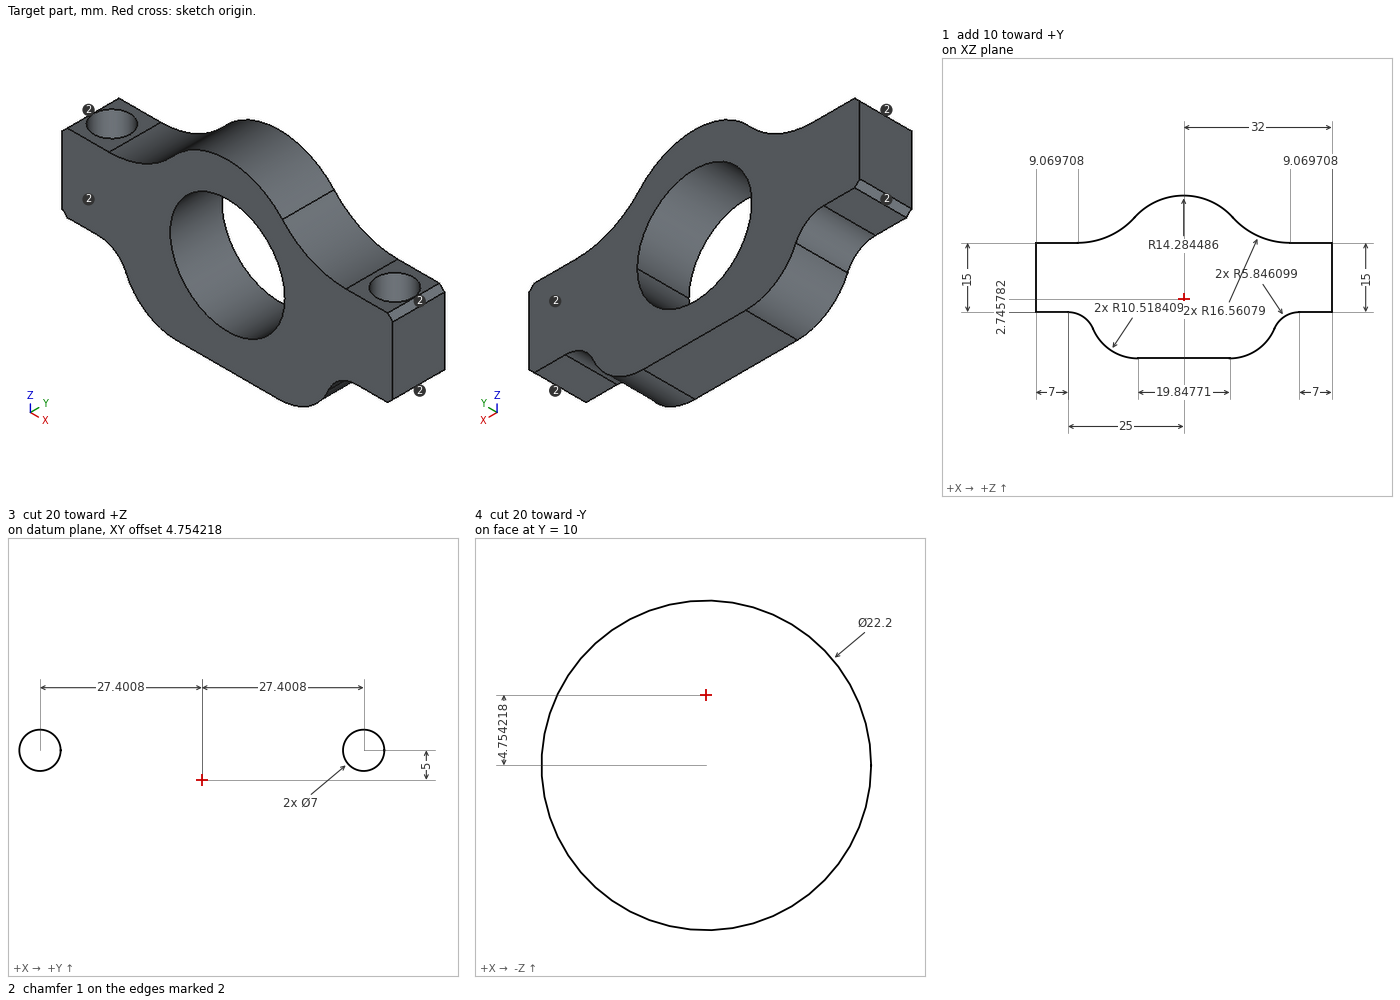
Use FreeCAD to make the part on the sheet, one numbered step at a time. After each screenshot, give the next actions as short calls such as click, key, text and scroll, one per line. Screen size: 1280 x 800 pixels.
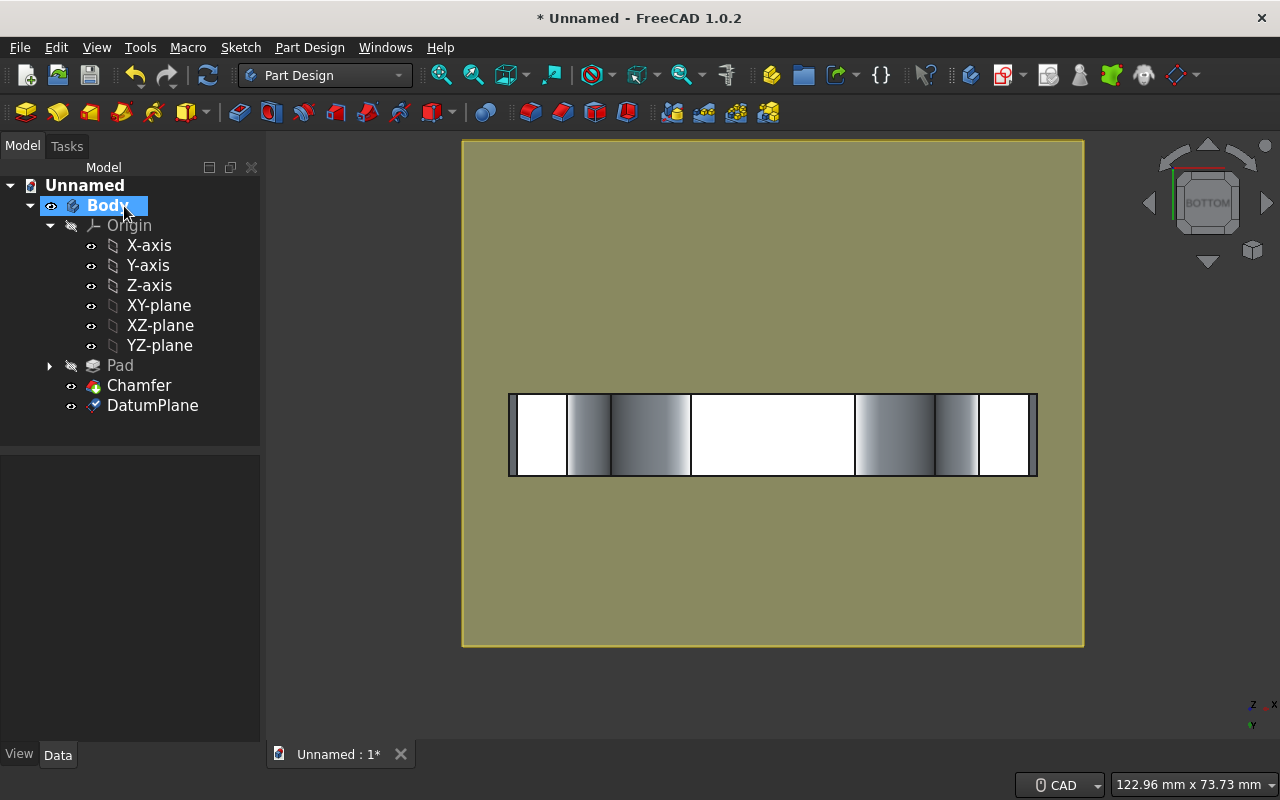
click(116, 406)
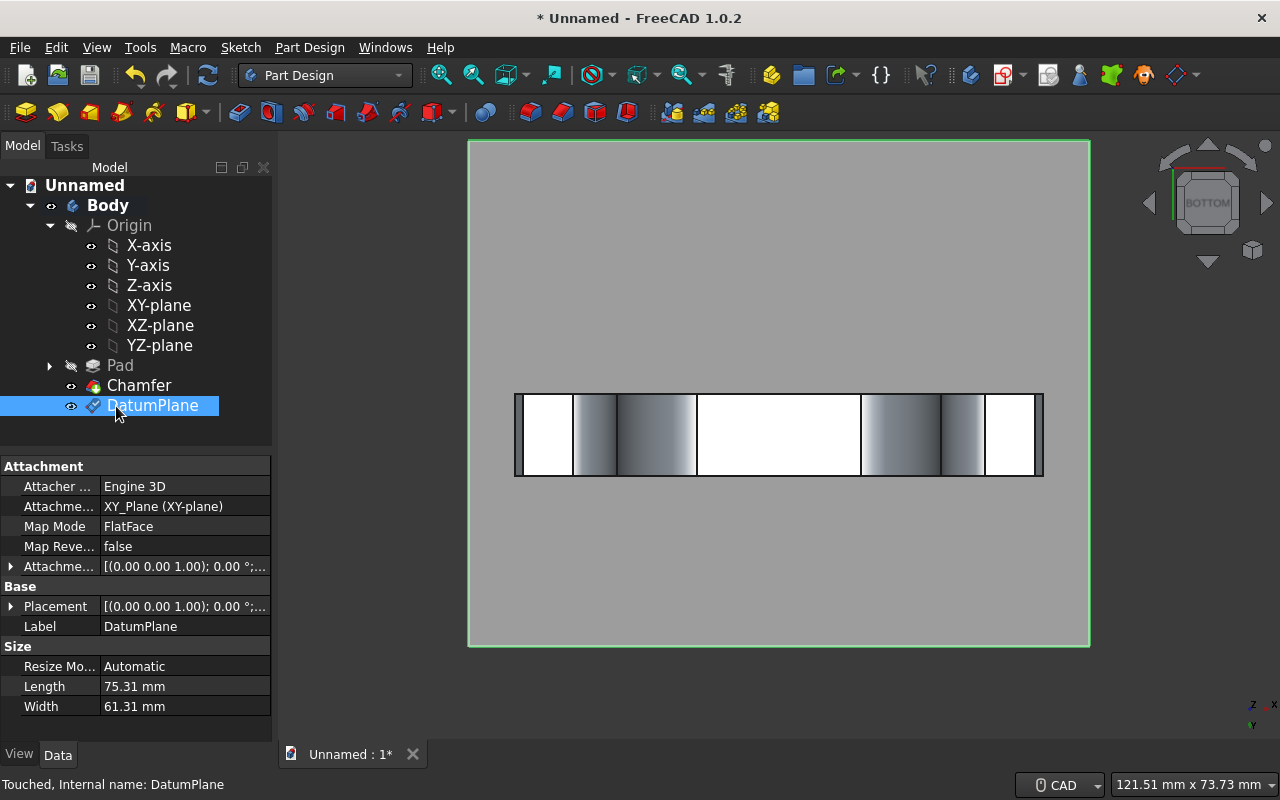
click(1004, 76)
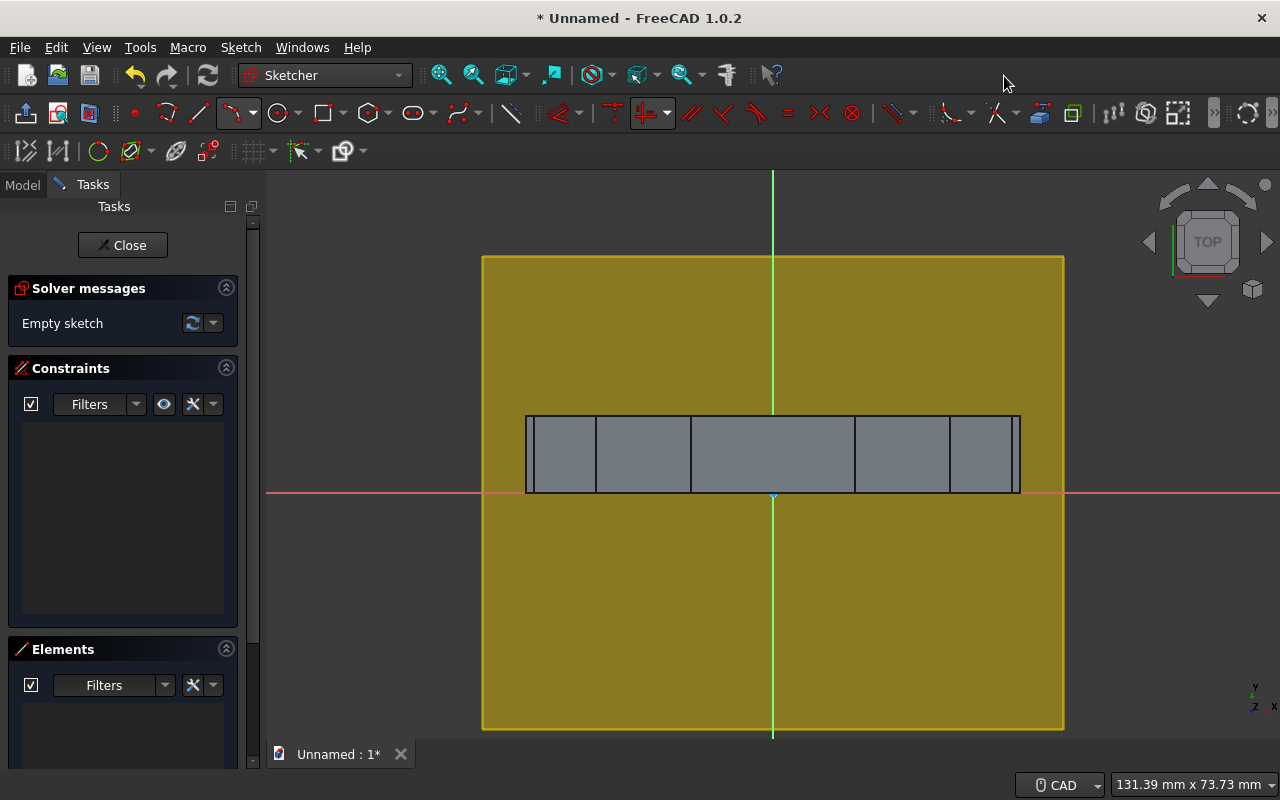
click(90, 114)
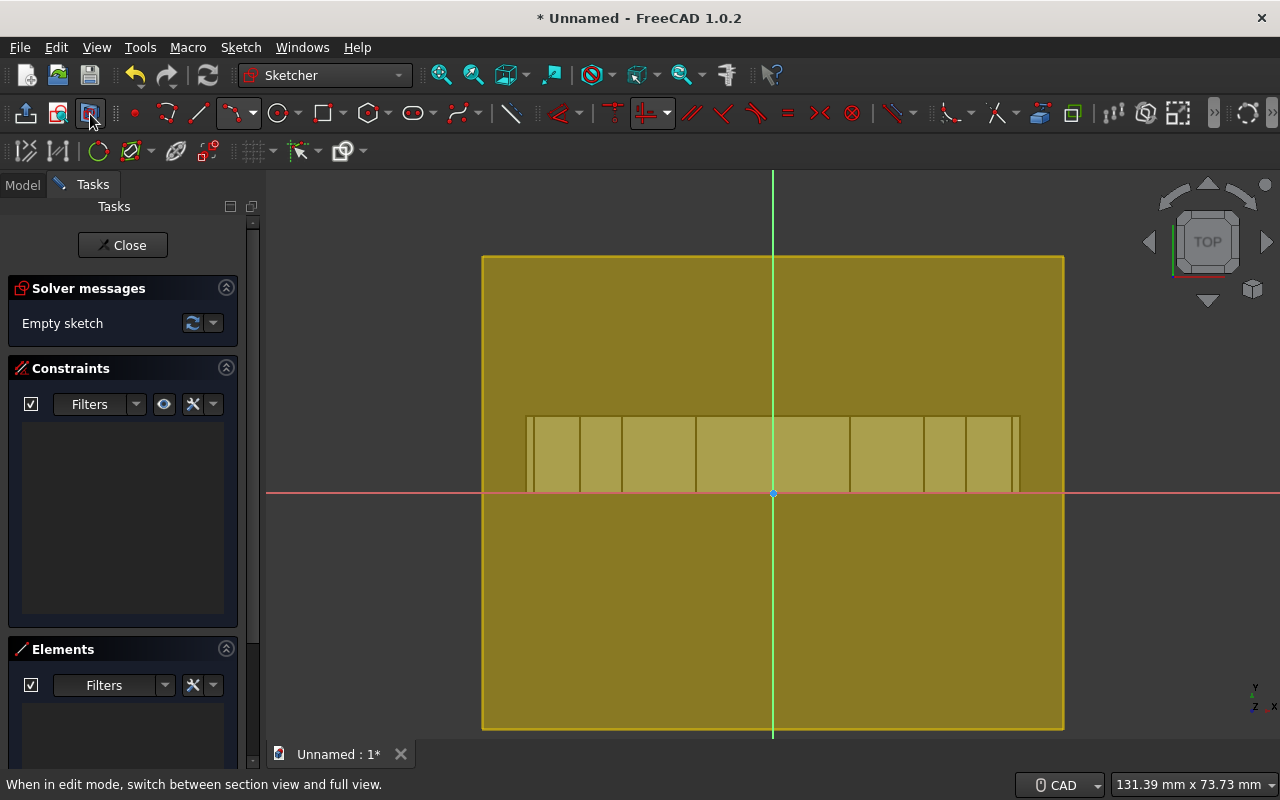
click(278, 114)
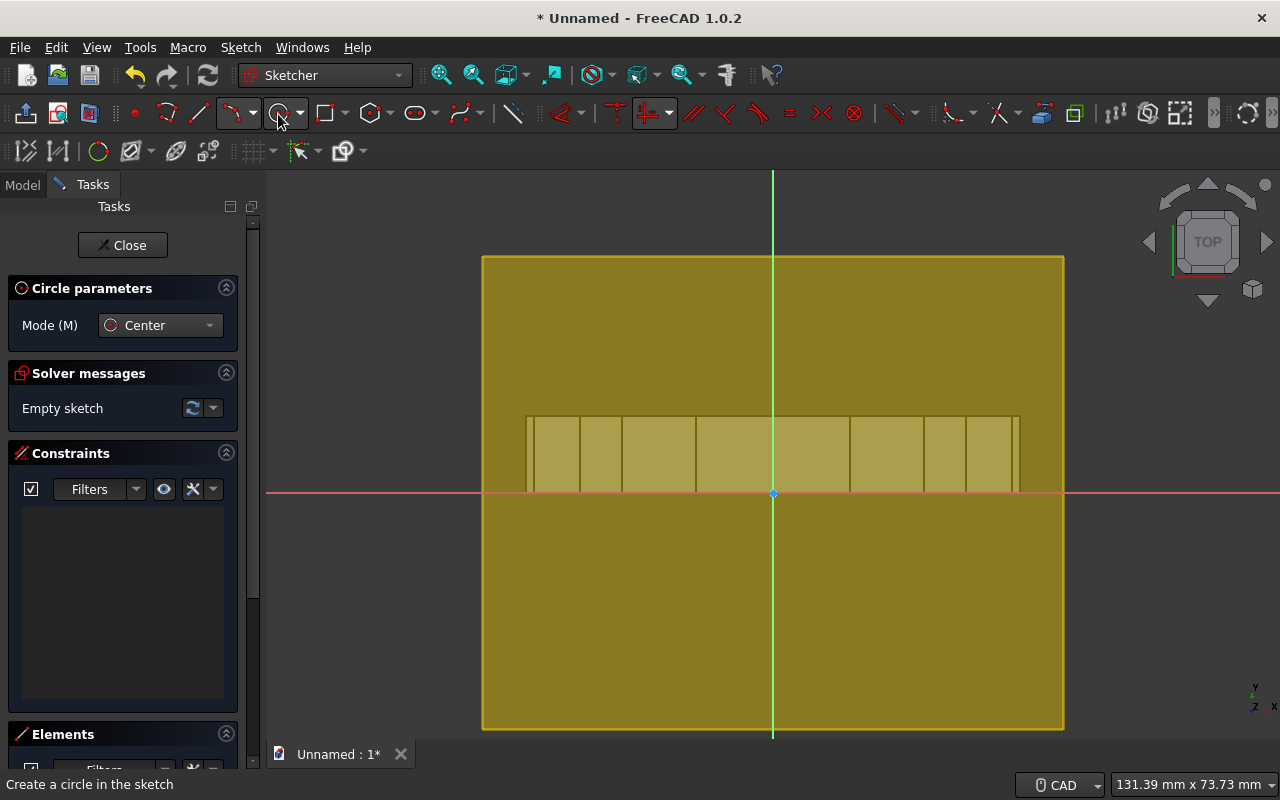
click(984, 454)
move(1004, 435)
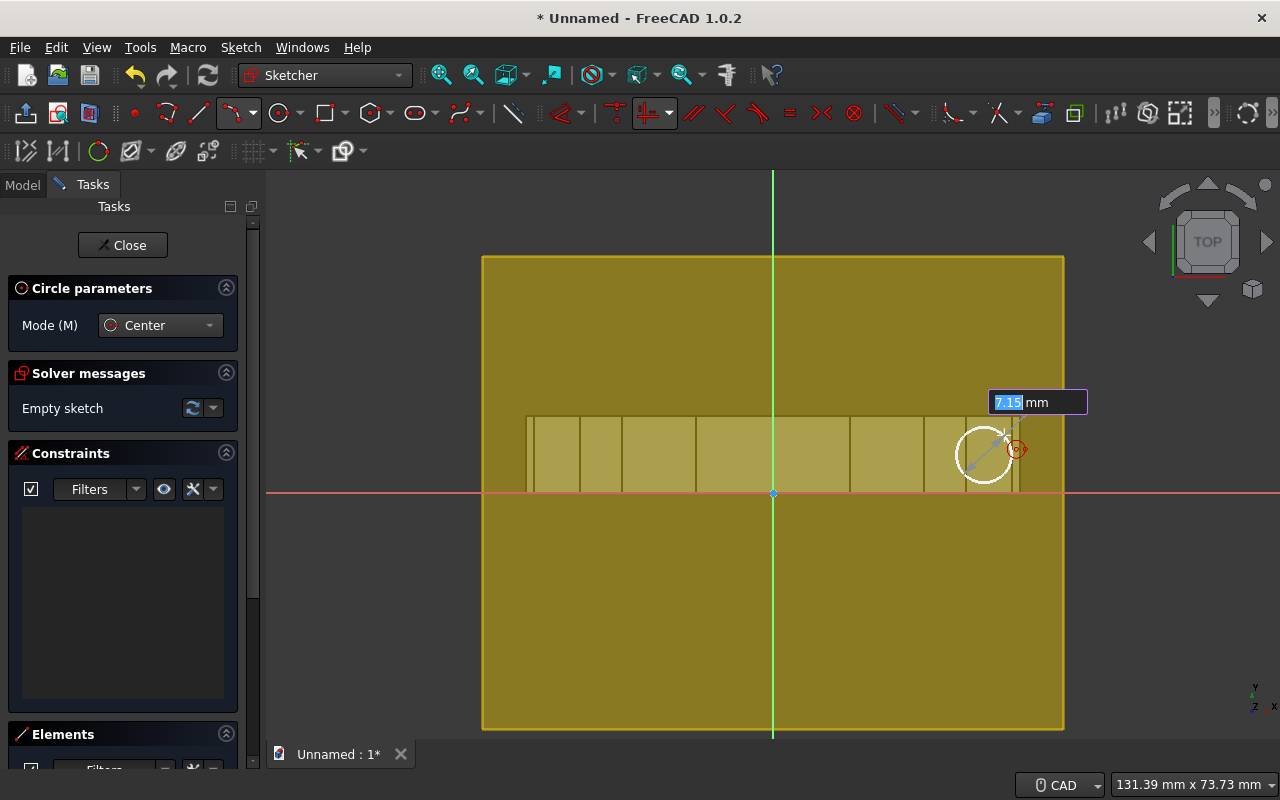
text(7)
key(Return)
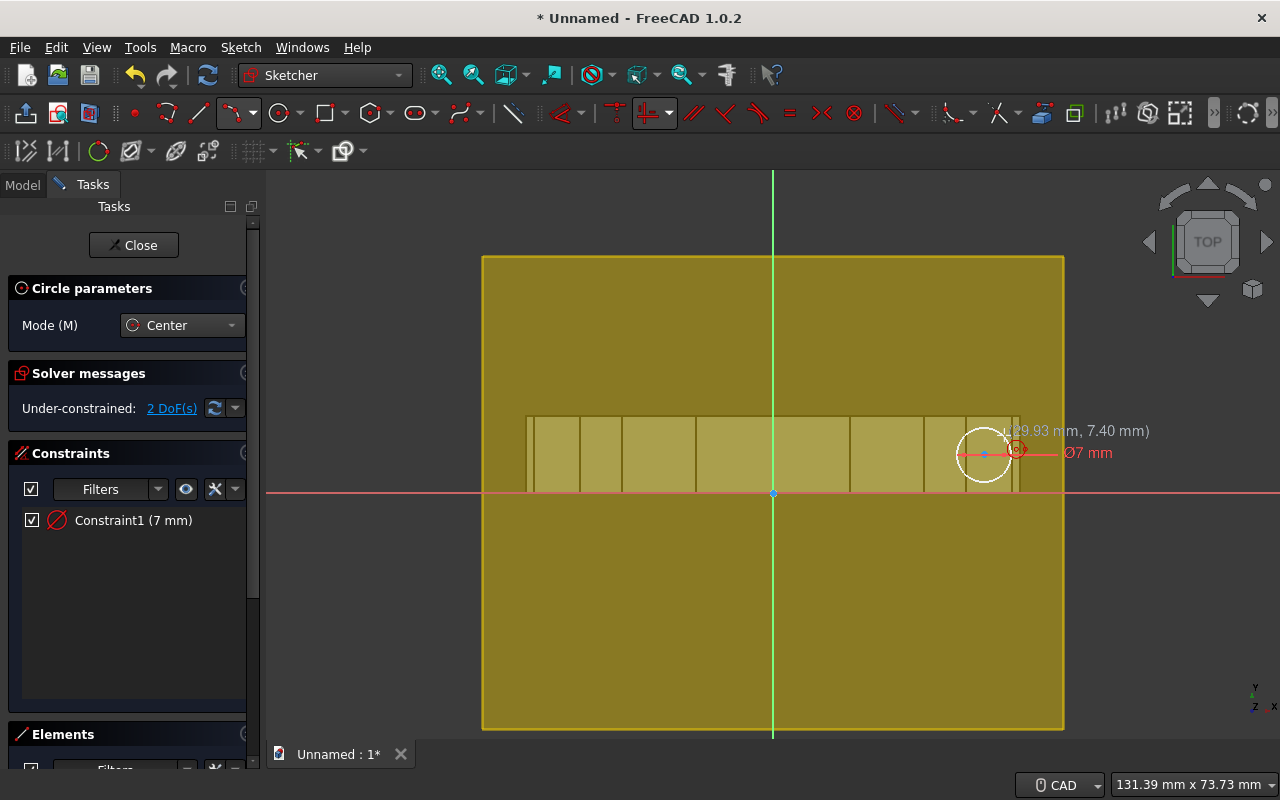
click(562, 454)
move(581, 435)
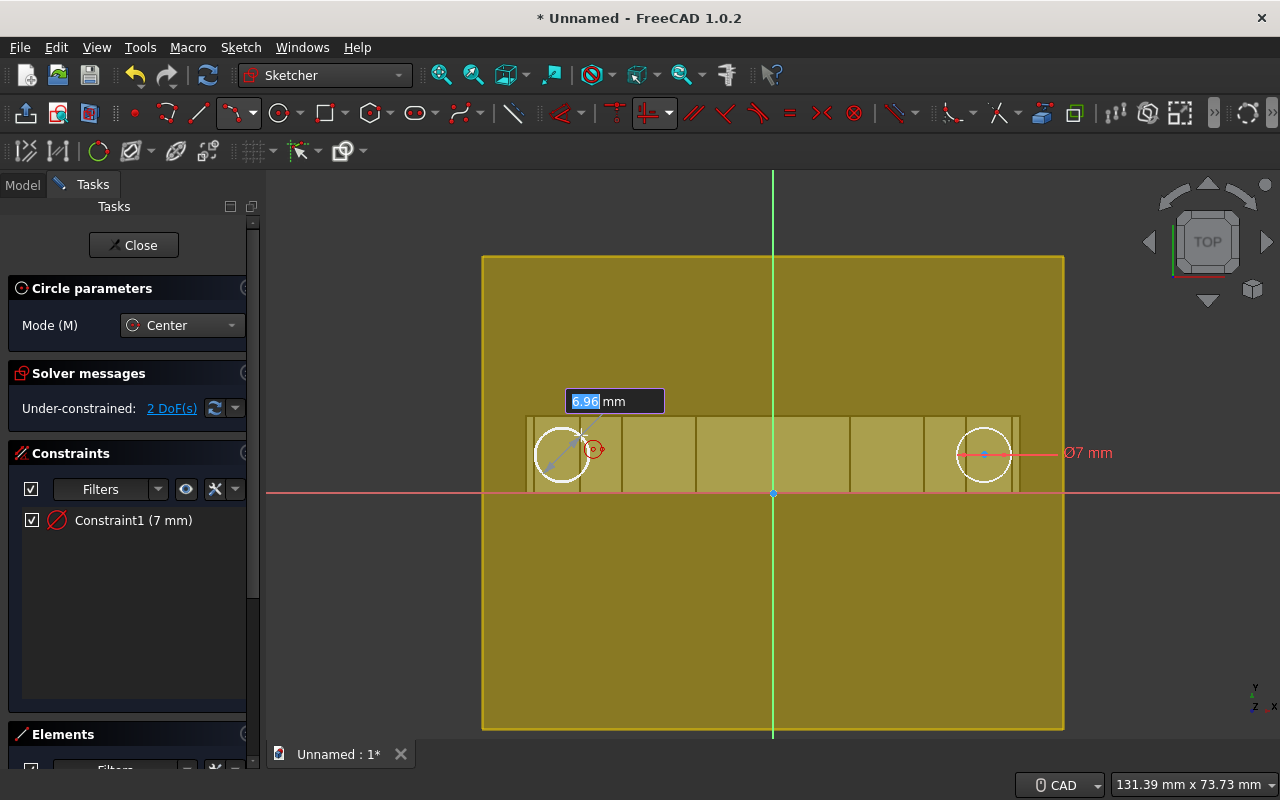
text(7)
key(Return)
key(Escape)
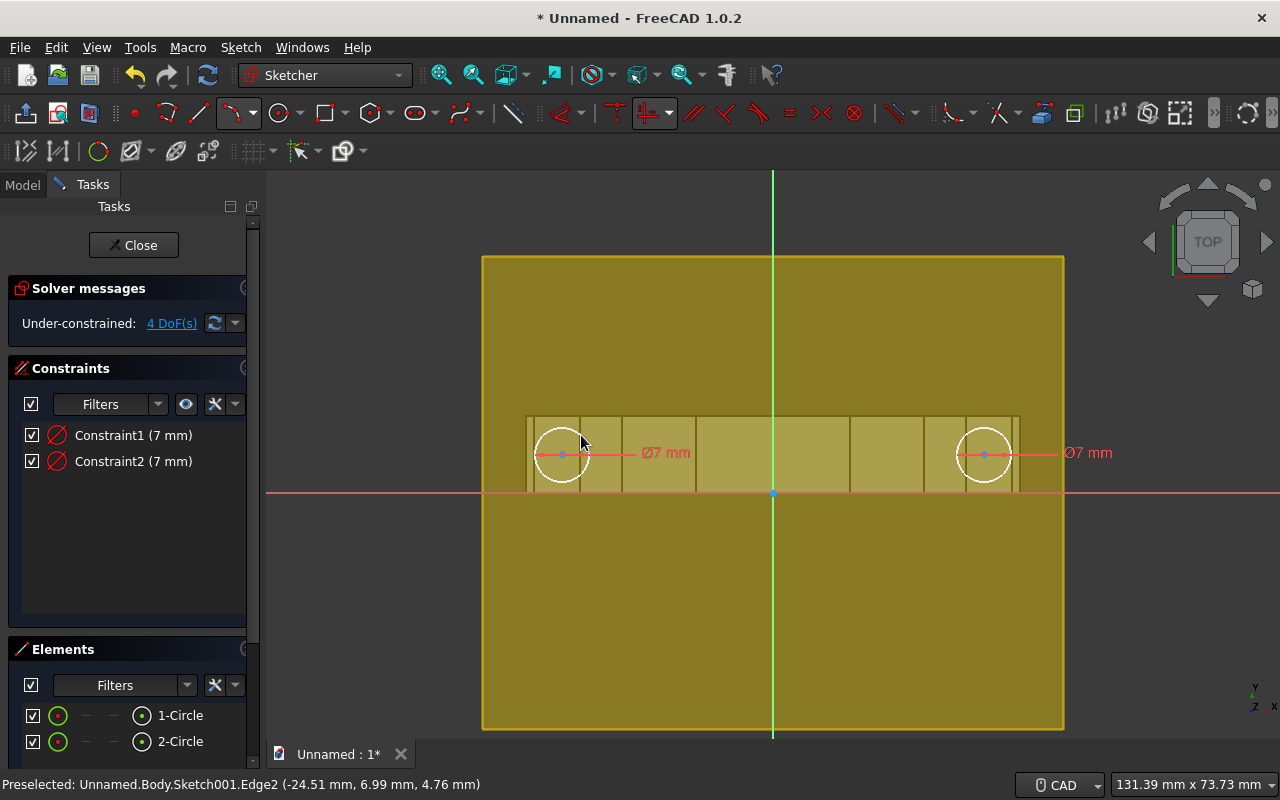
click(984, 455)